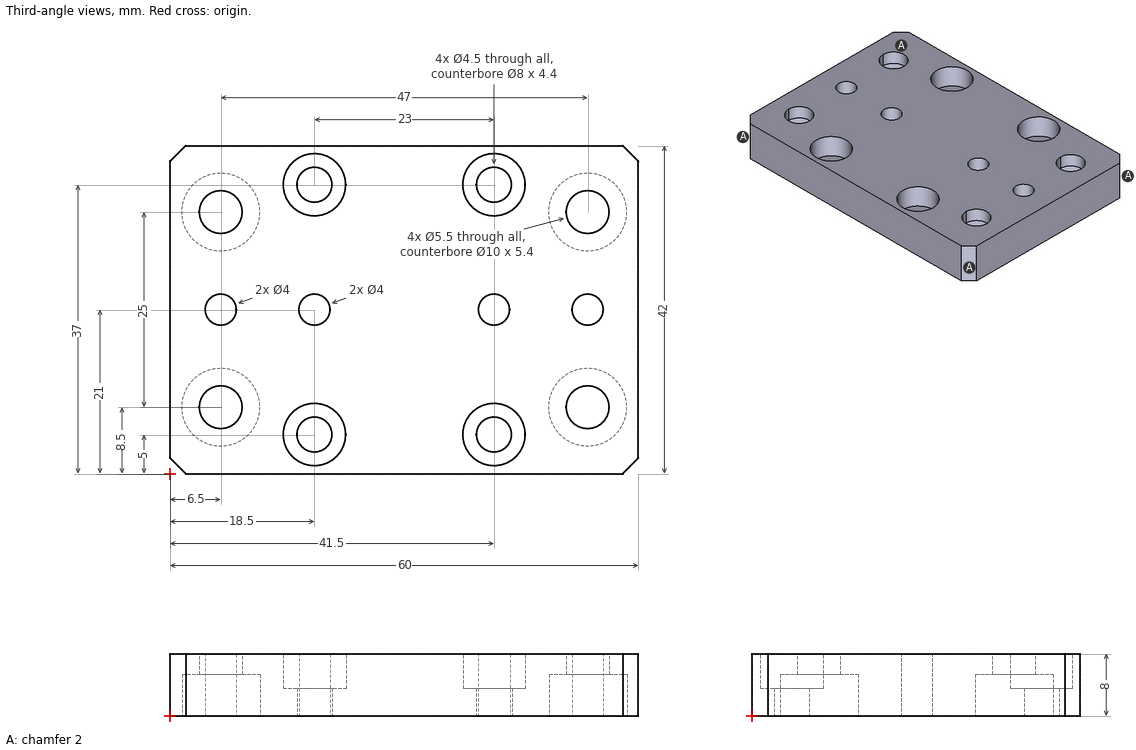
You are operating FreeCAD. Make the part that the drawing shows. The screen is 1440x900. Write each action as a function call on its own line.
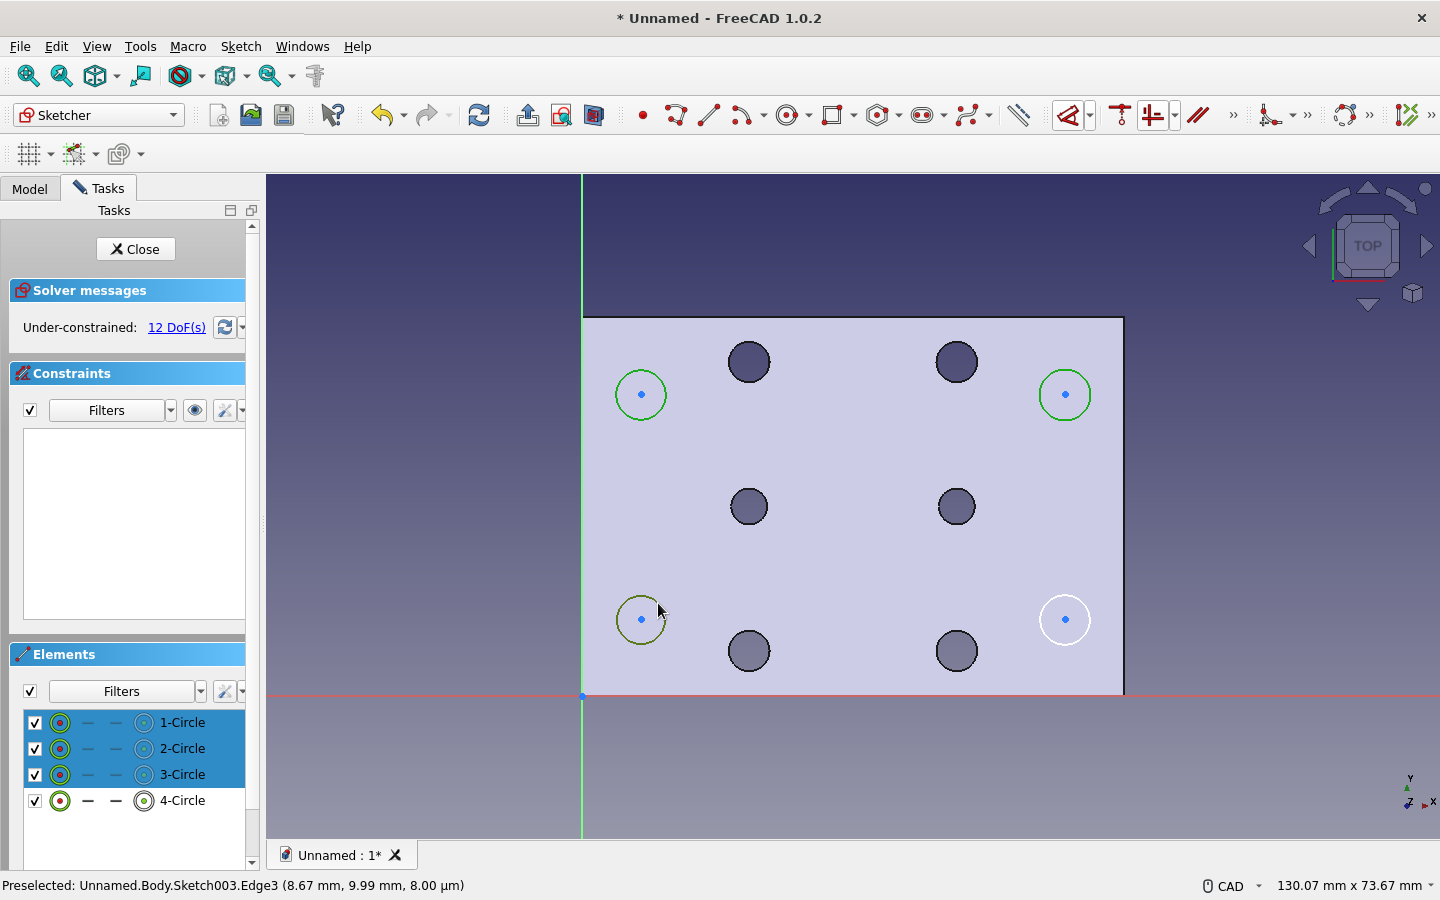
click(1082, 602)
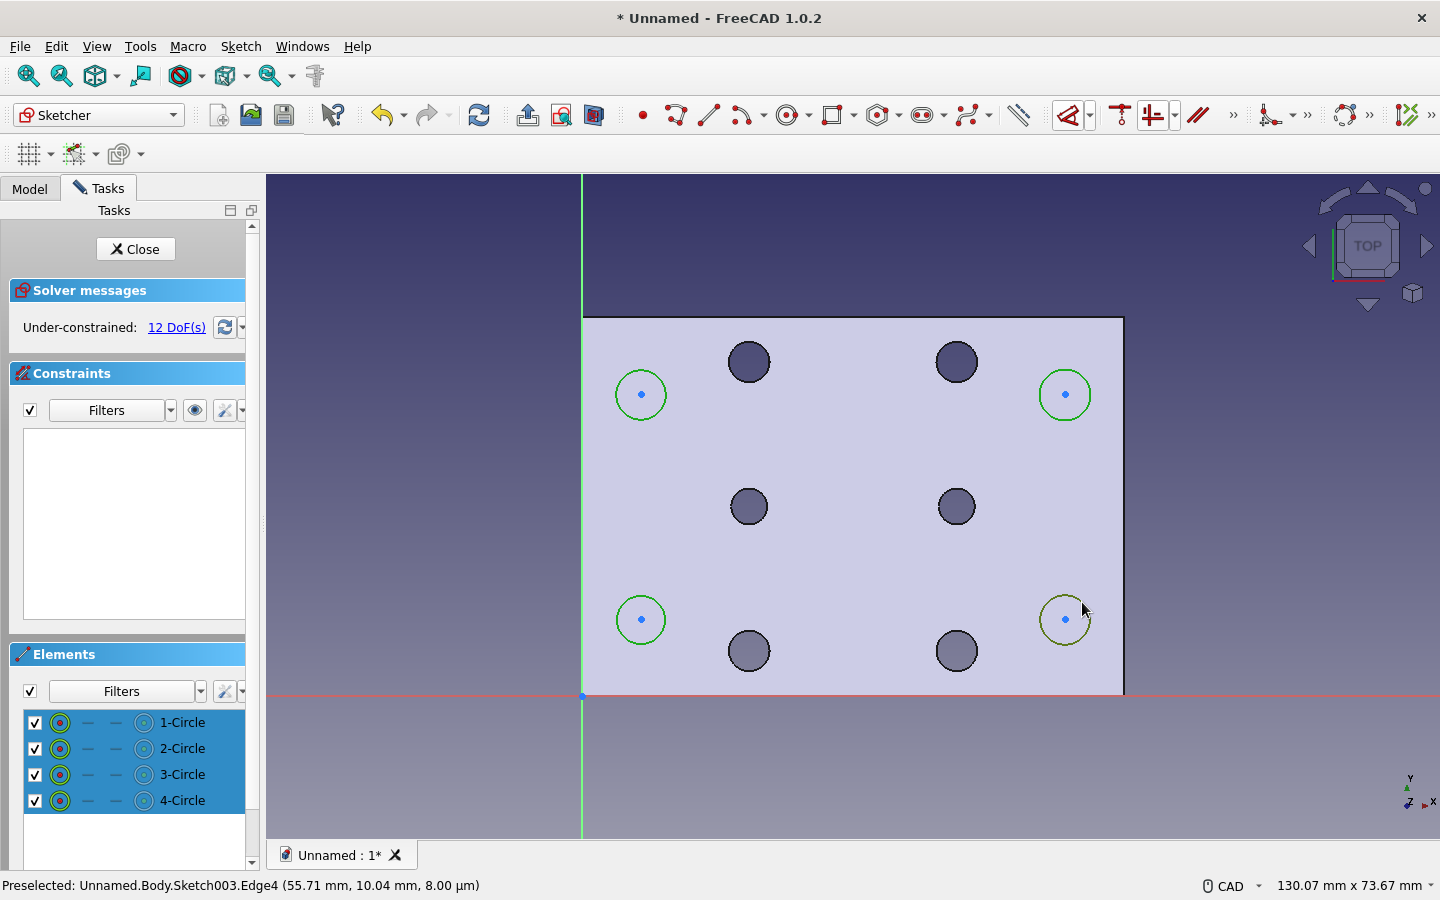
key(e)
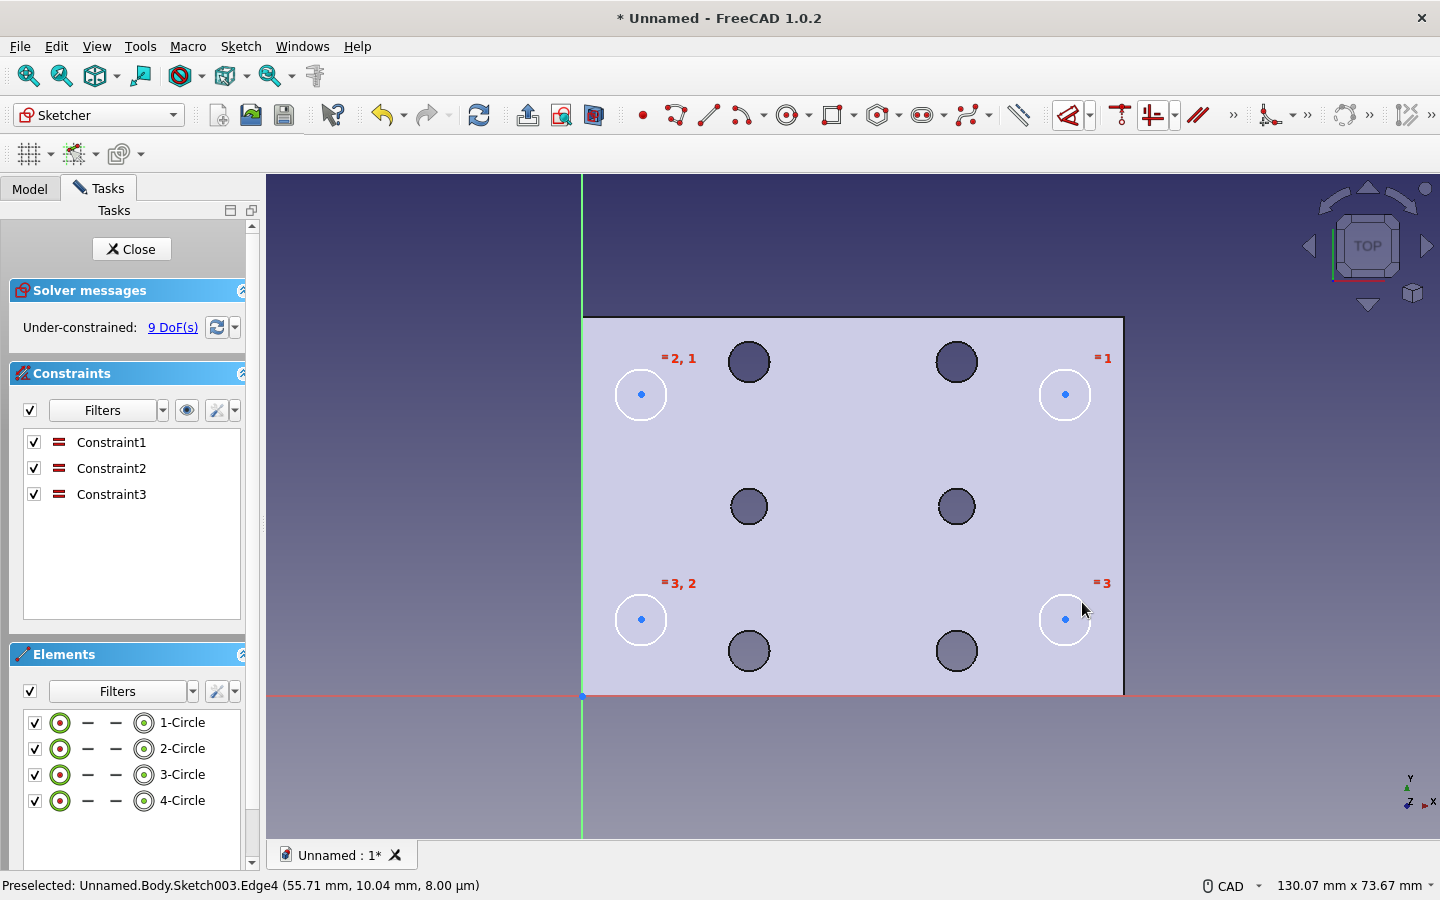
click(1065, 395)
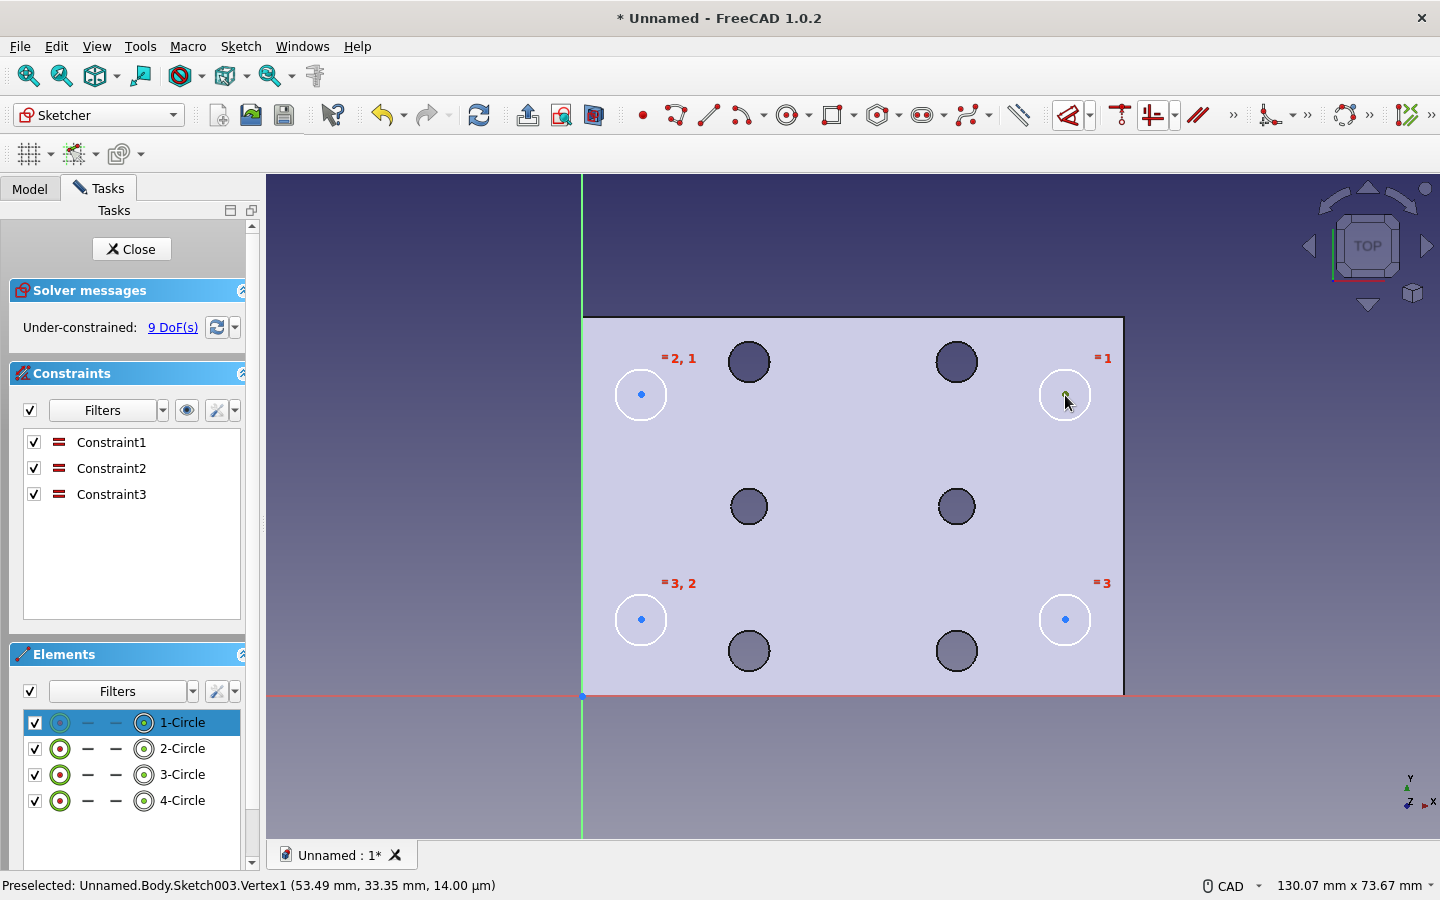
click(641, 395)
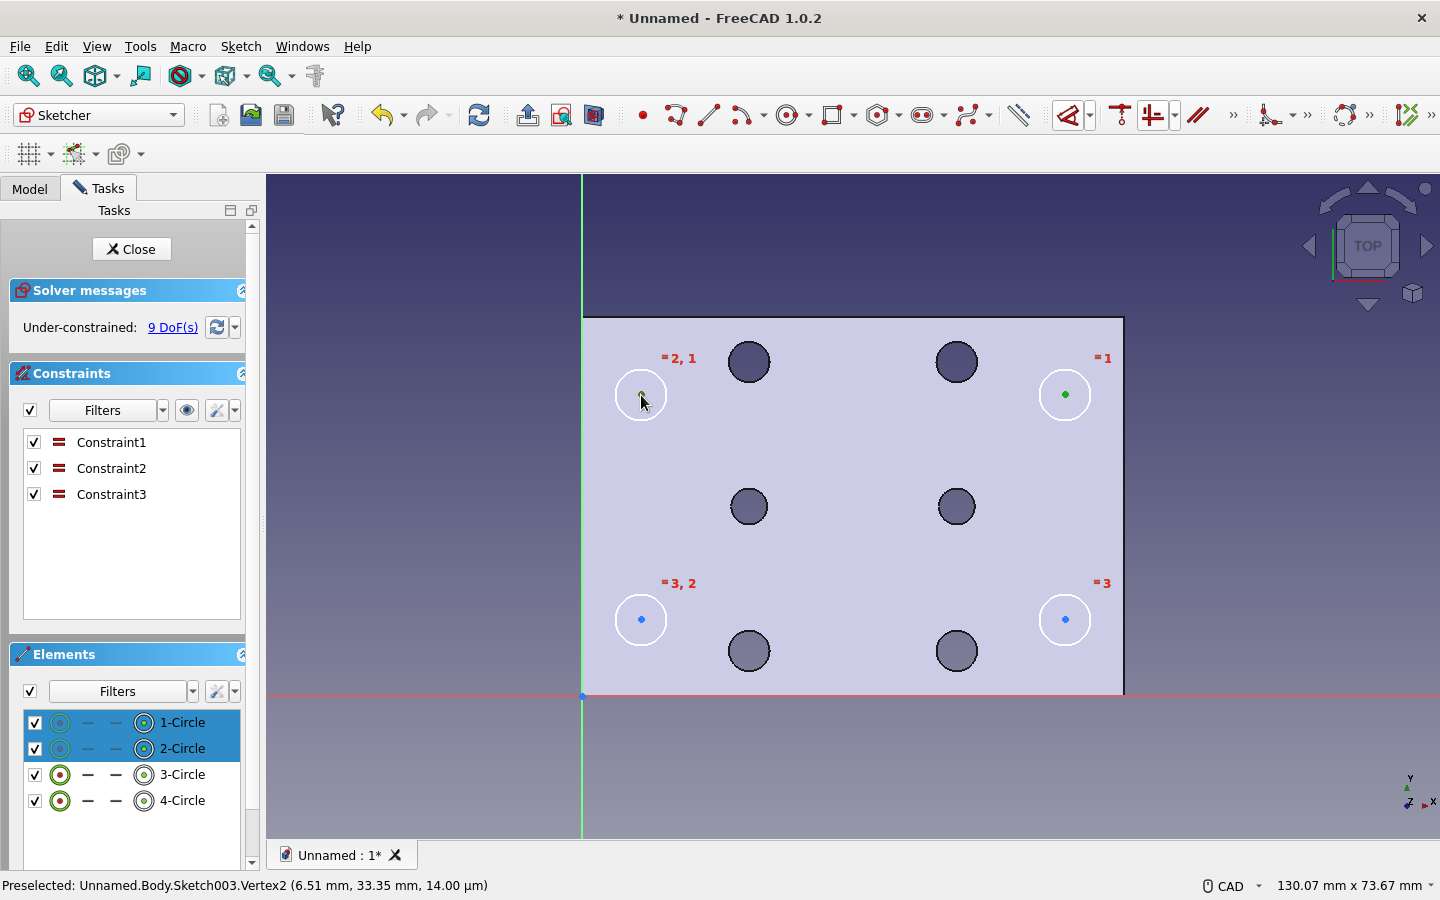
key(h)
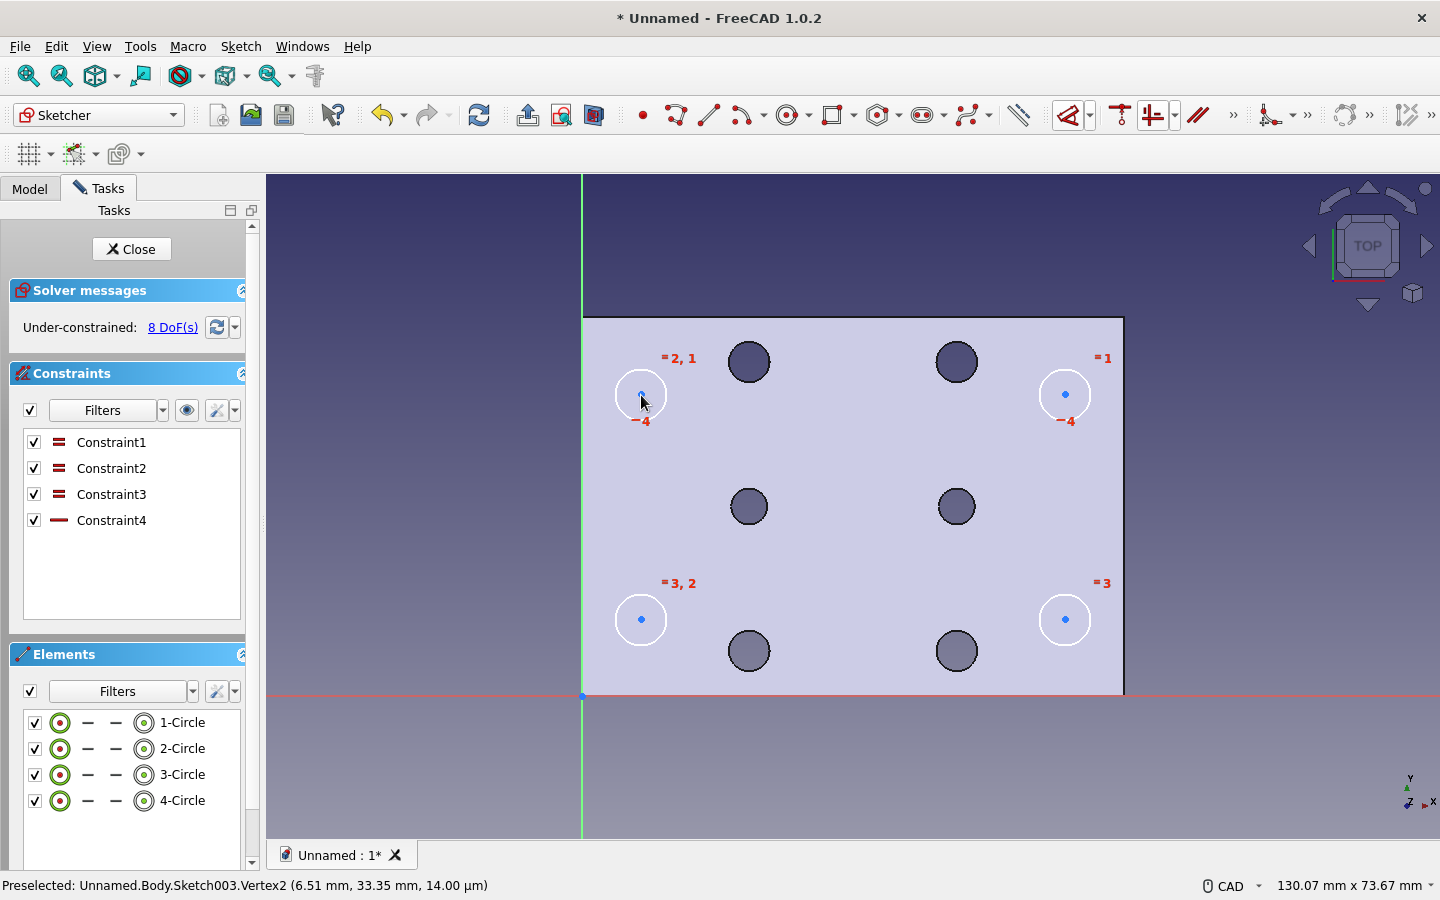
click(641, 395)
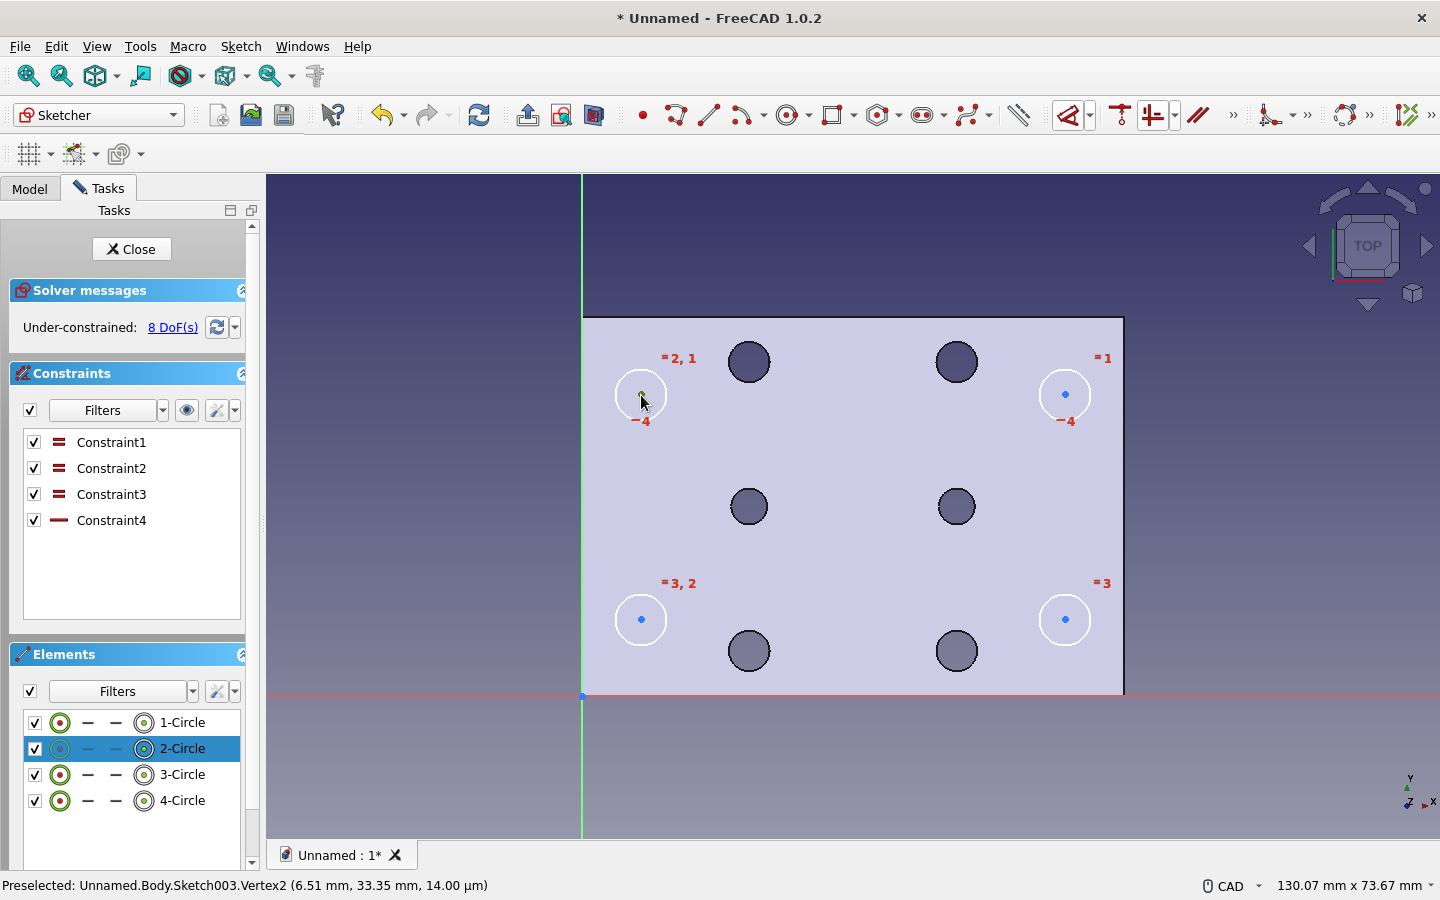
click(641, 620)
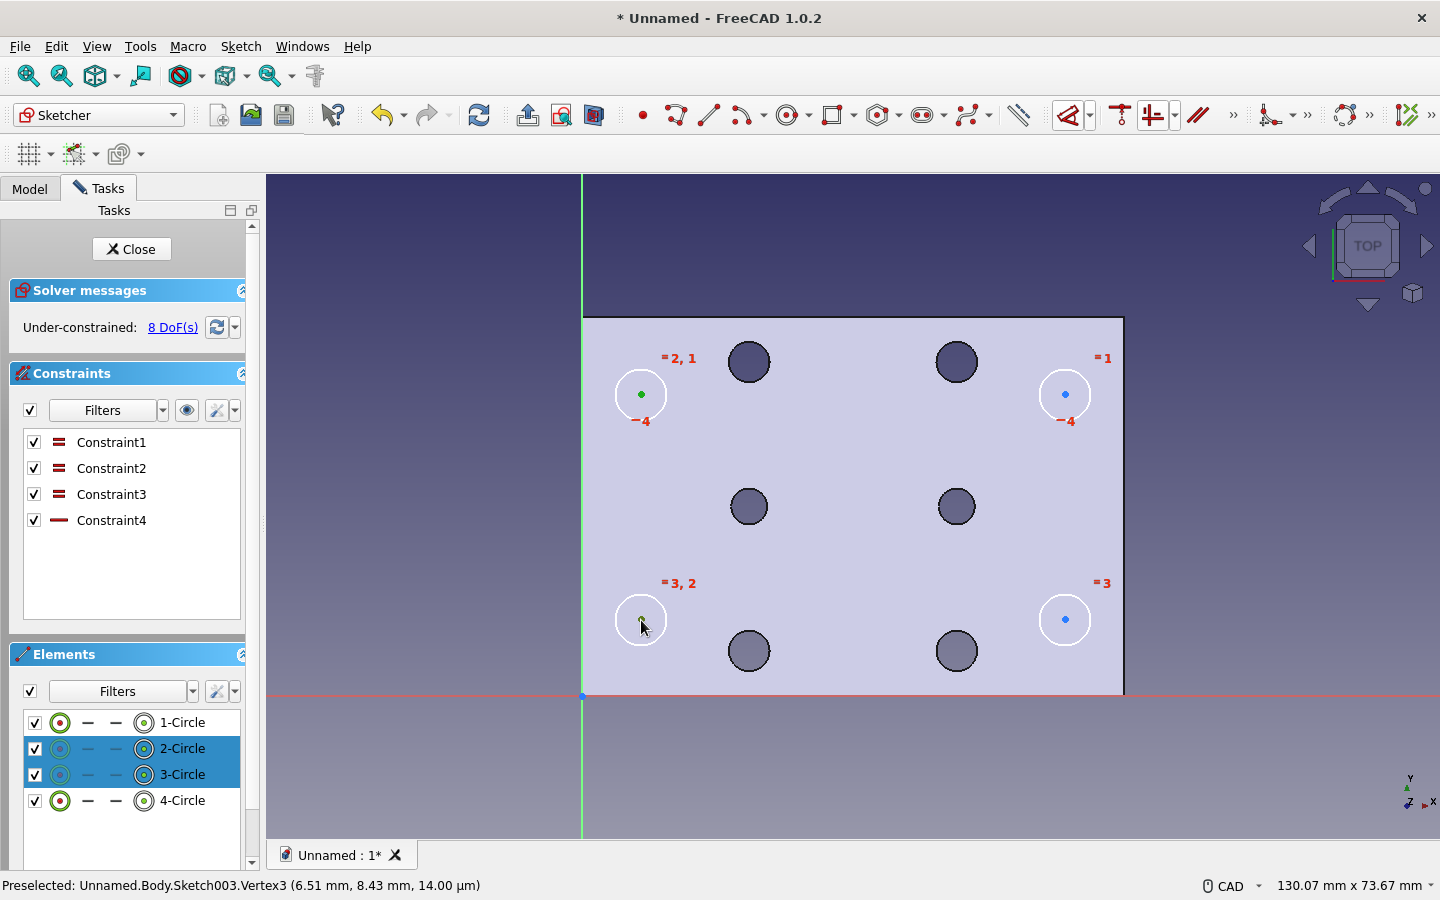
key(v)